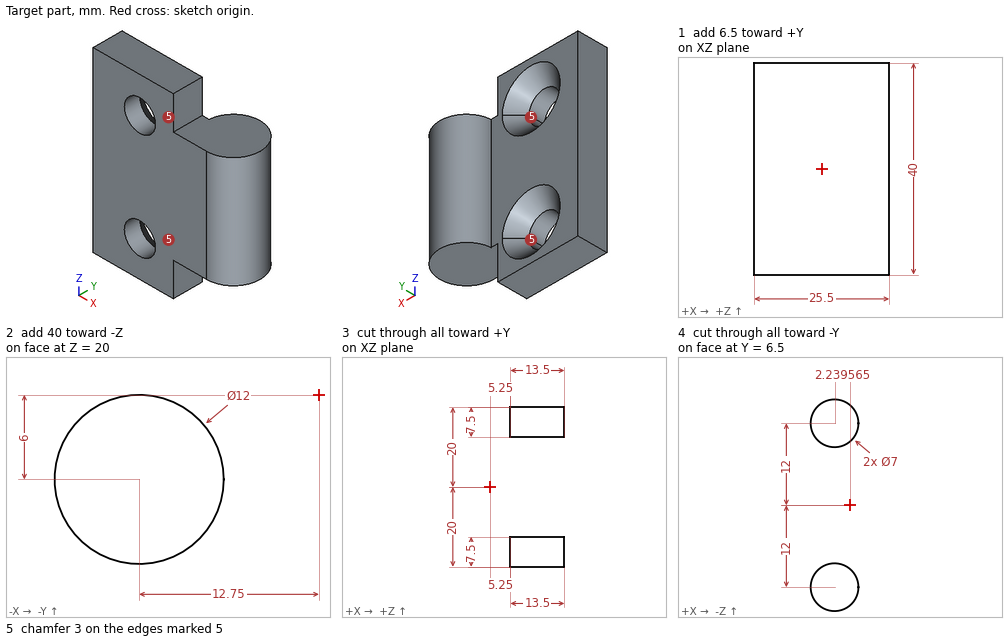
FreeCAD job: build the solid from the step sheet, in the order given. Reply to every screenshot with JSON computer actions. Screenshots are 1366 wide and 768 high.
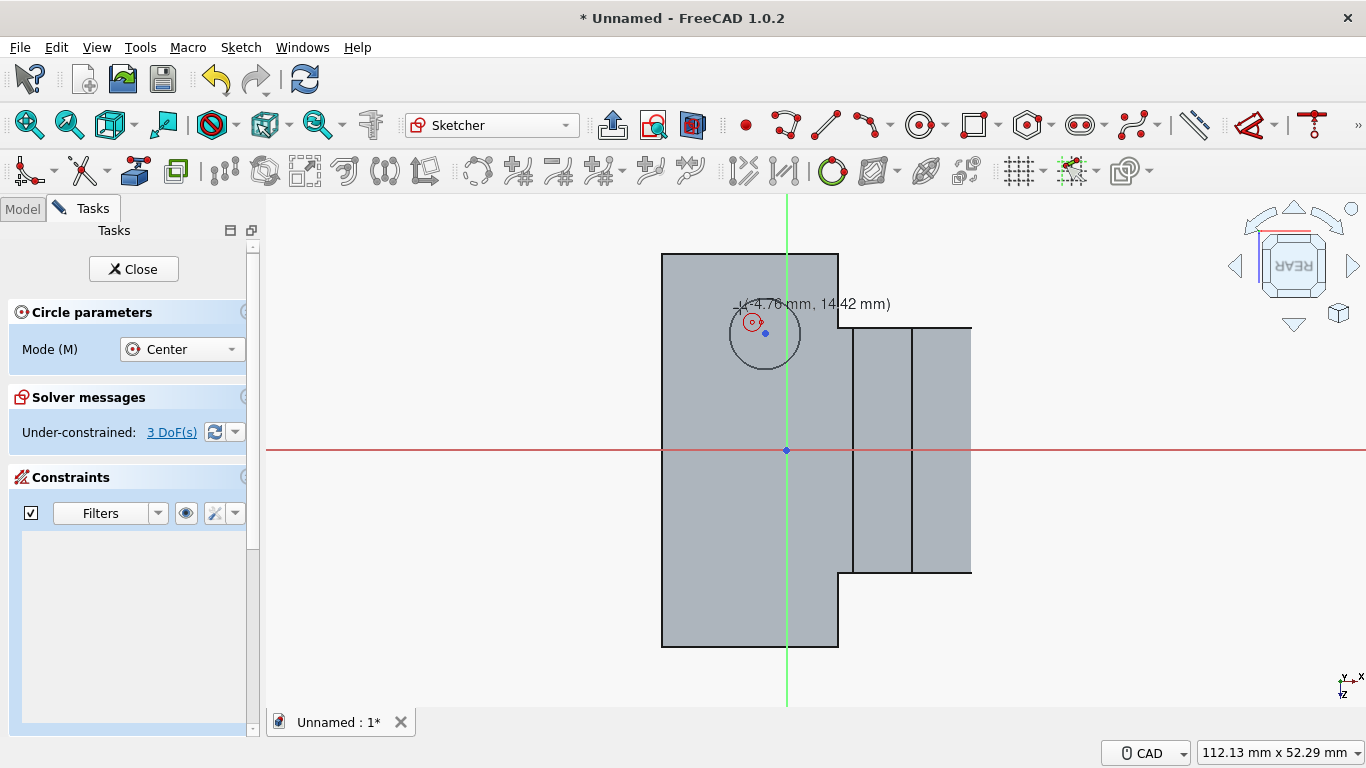
{"action": "left_click", "coordinate": [765, 568]}
{"action": "left_click", "coordinate": [740, 544]}
{"action": "key", "text": "Escape"}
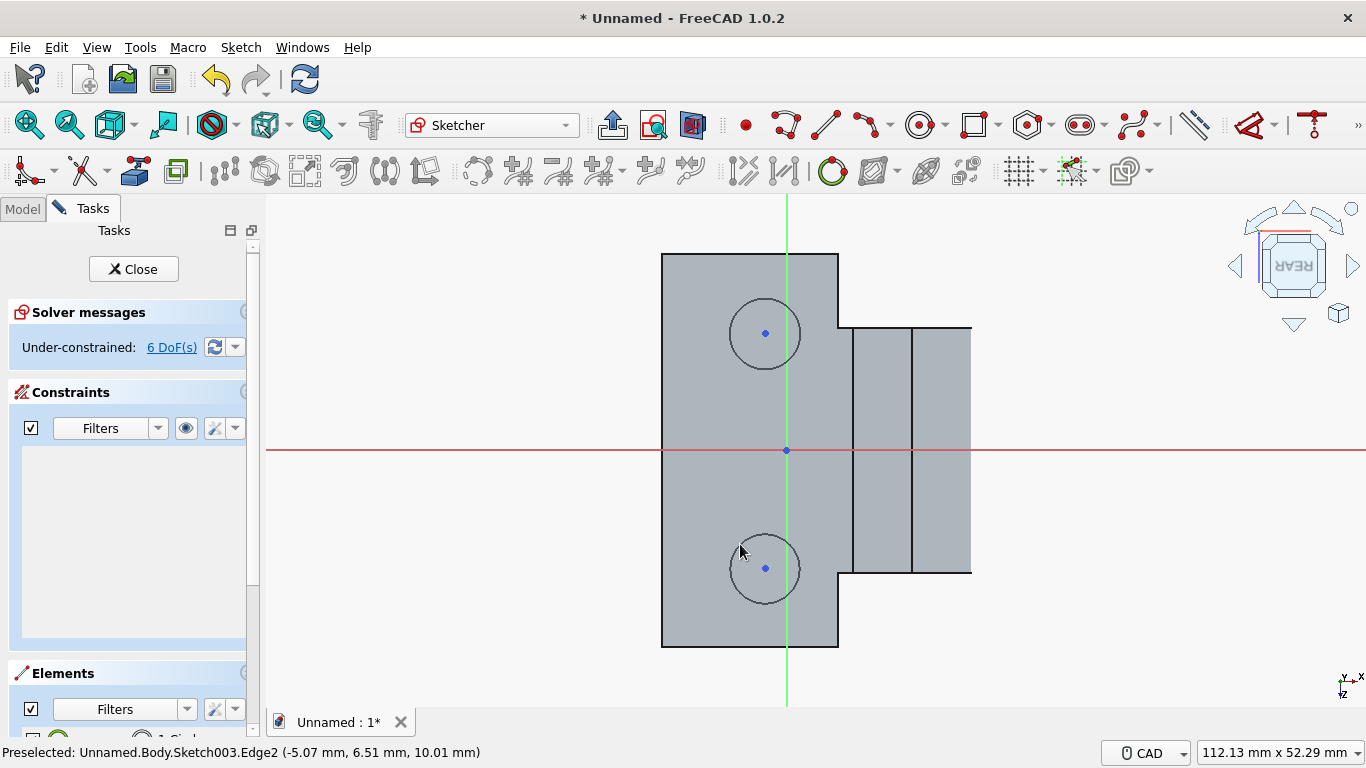
{"action": "left_click", "coordinate": [790, 309]}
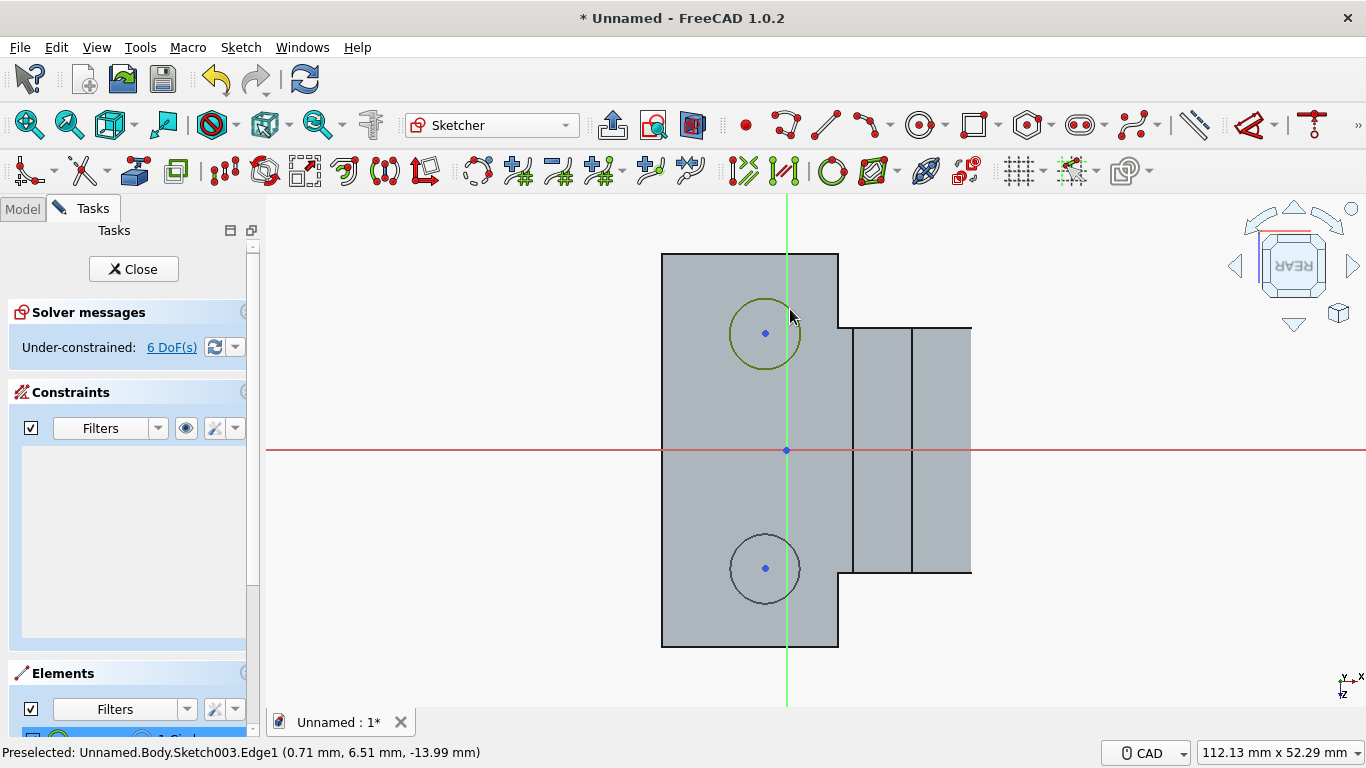
{"action": "left_click", "coordinate": [789, 544]}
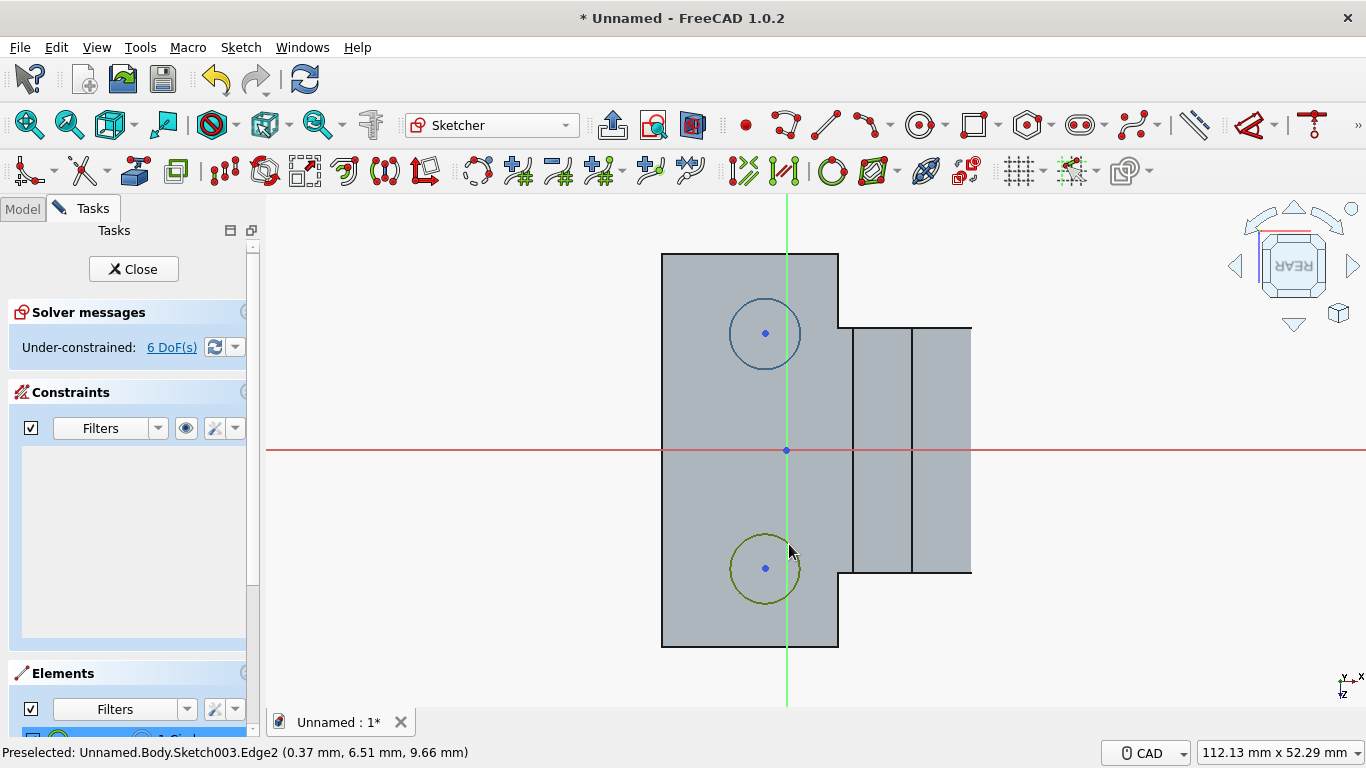
{"action": "key", "text": "e"}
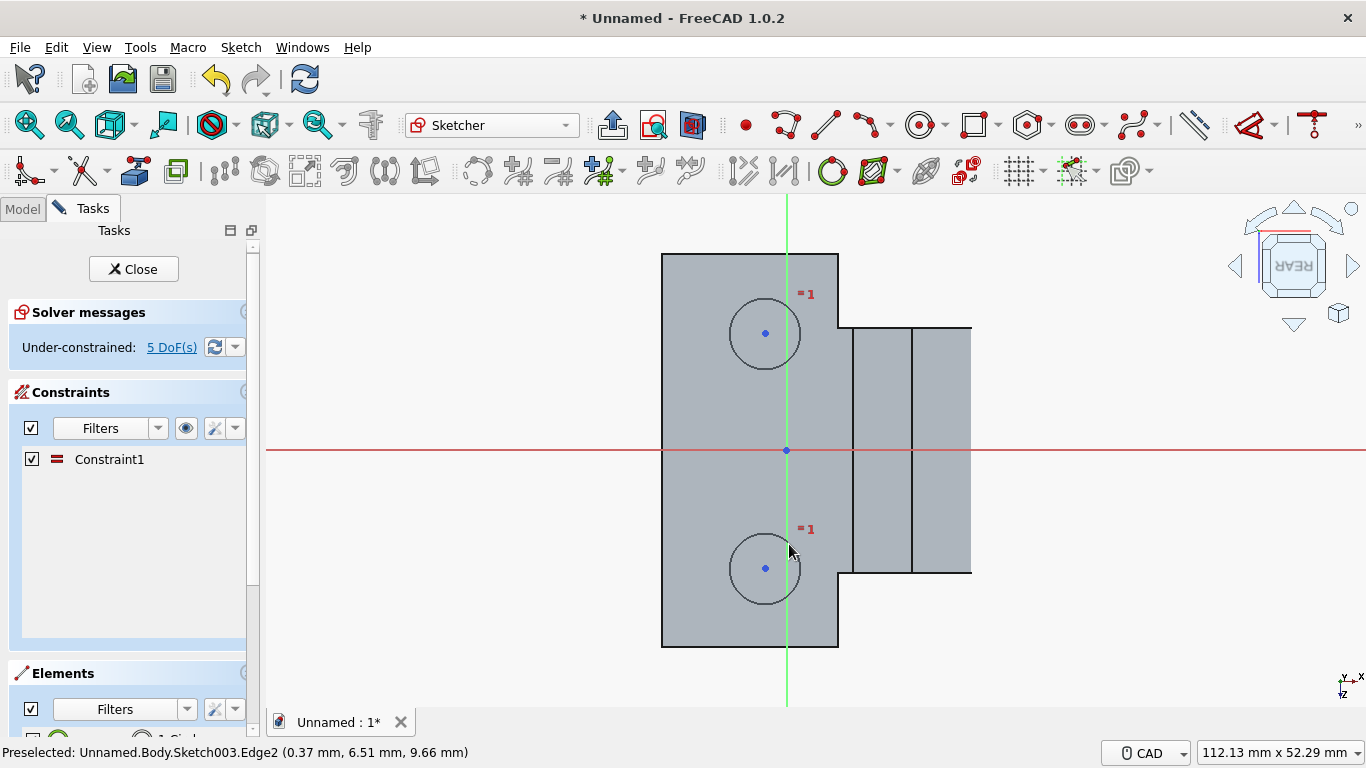
{"action": "left_click", "coordinate": [765, 334]}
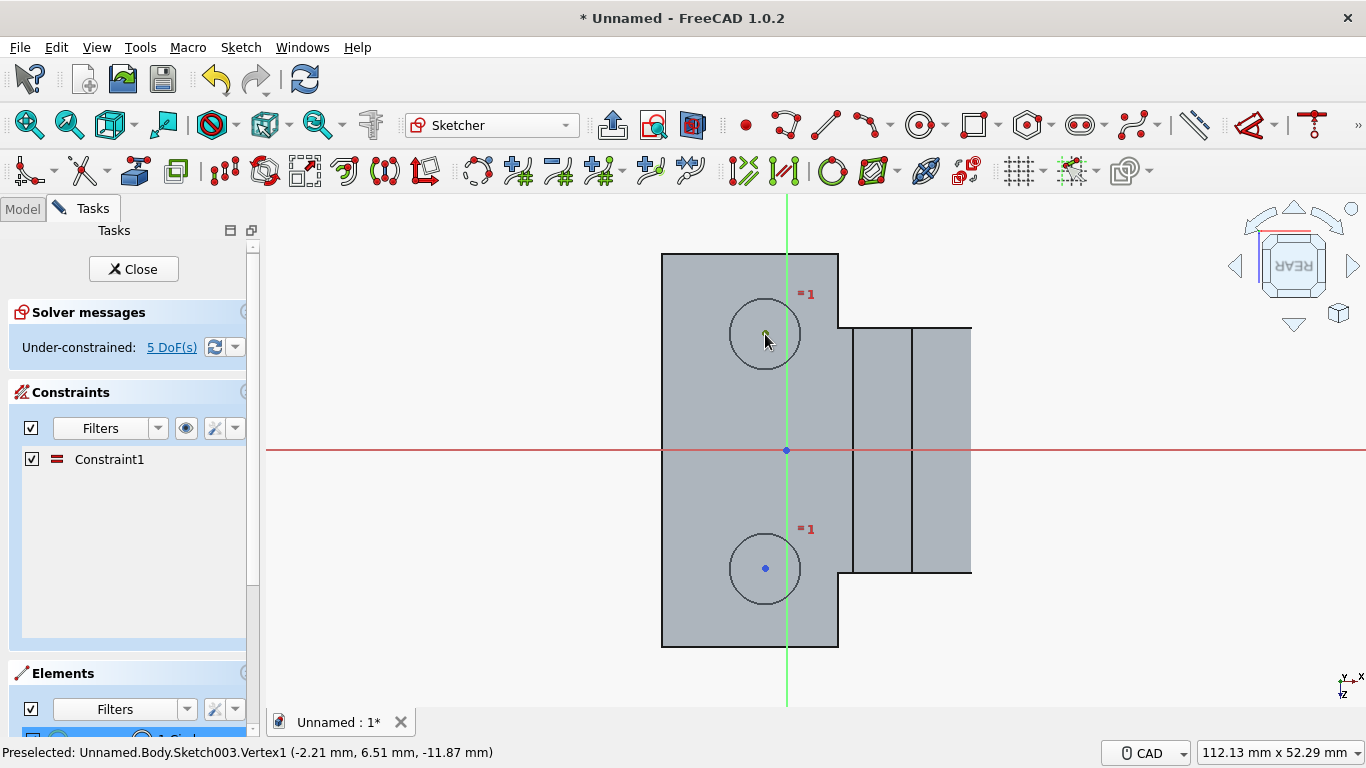
{"action": "left_click", "coordinate": [765, 569]}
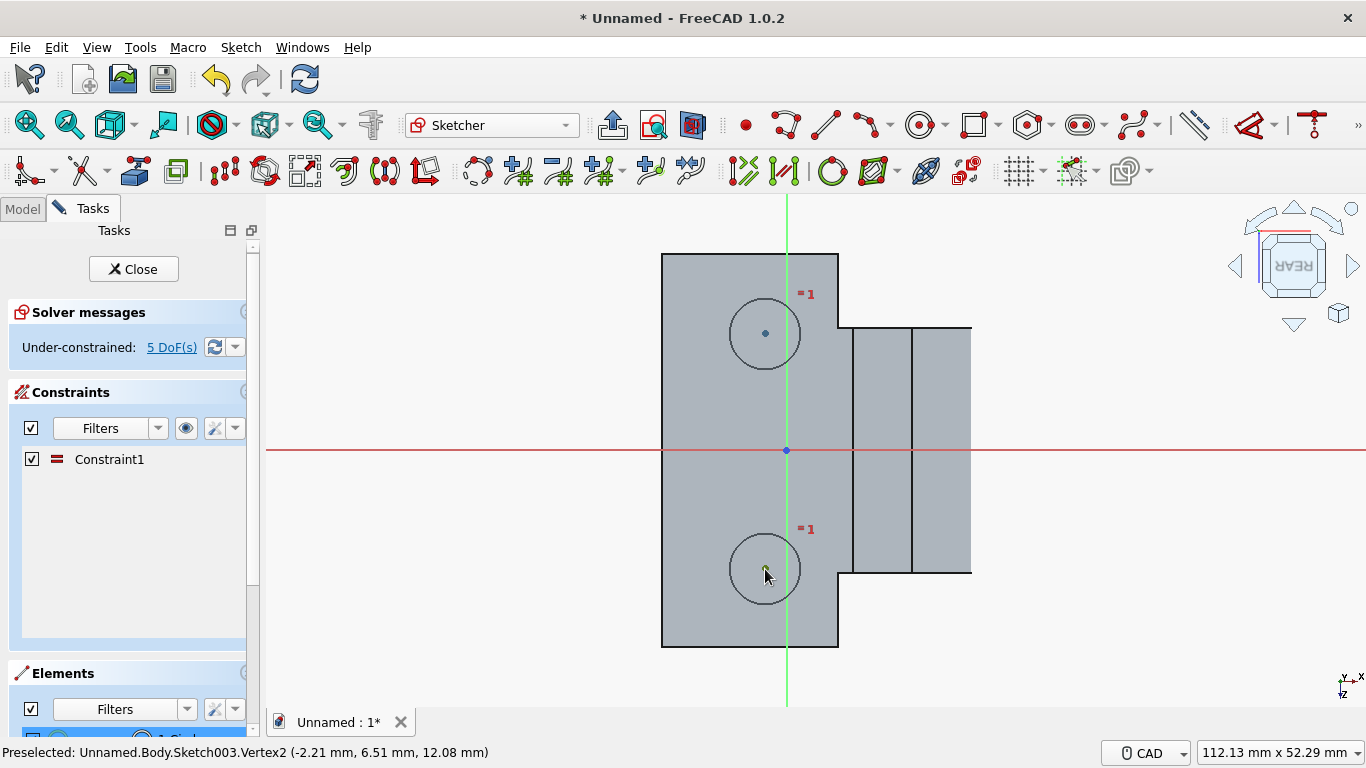
{"action": "key", "text": "v"}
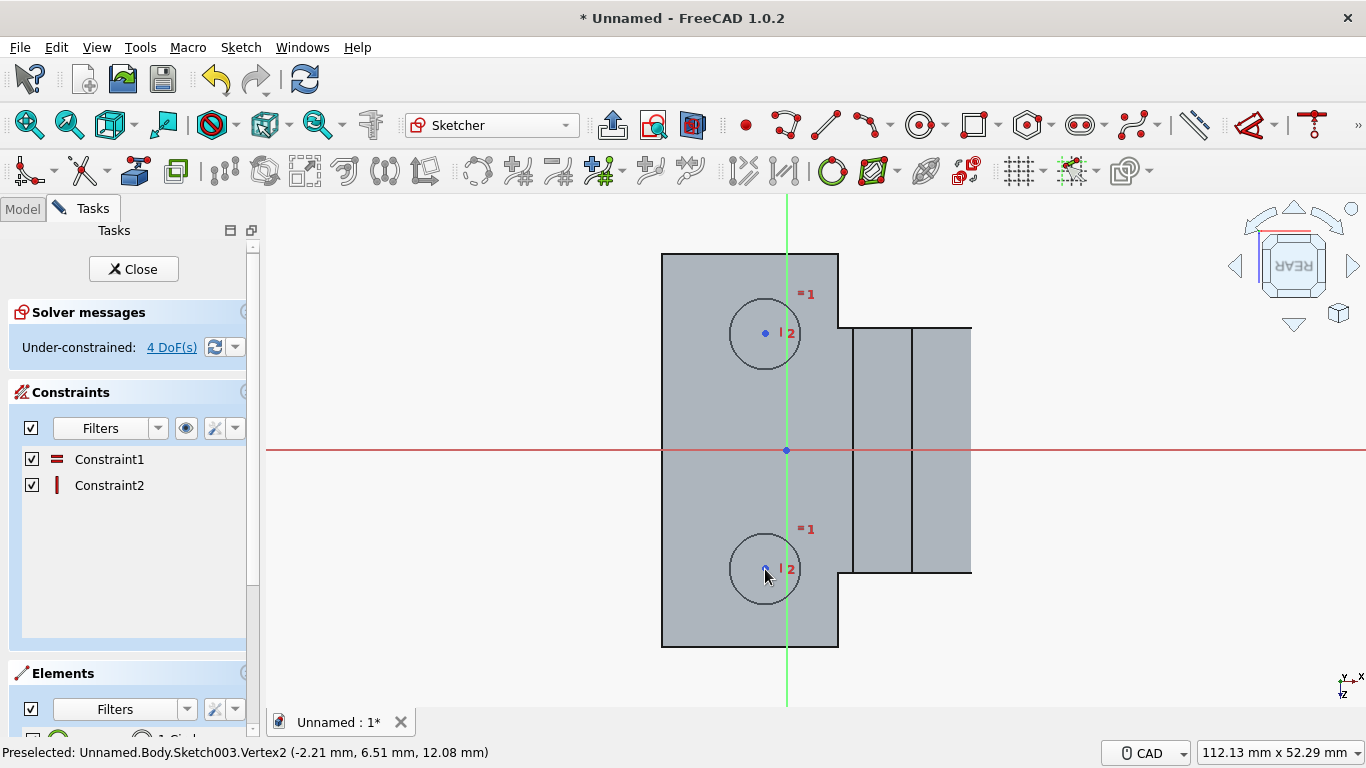
{"action": "key", "text": "d"}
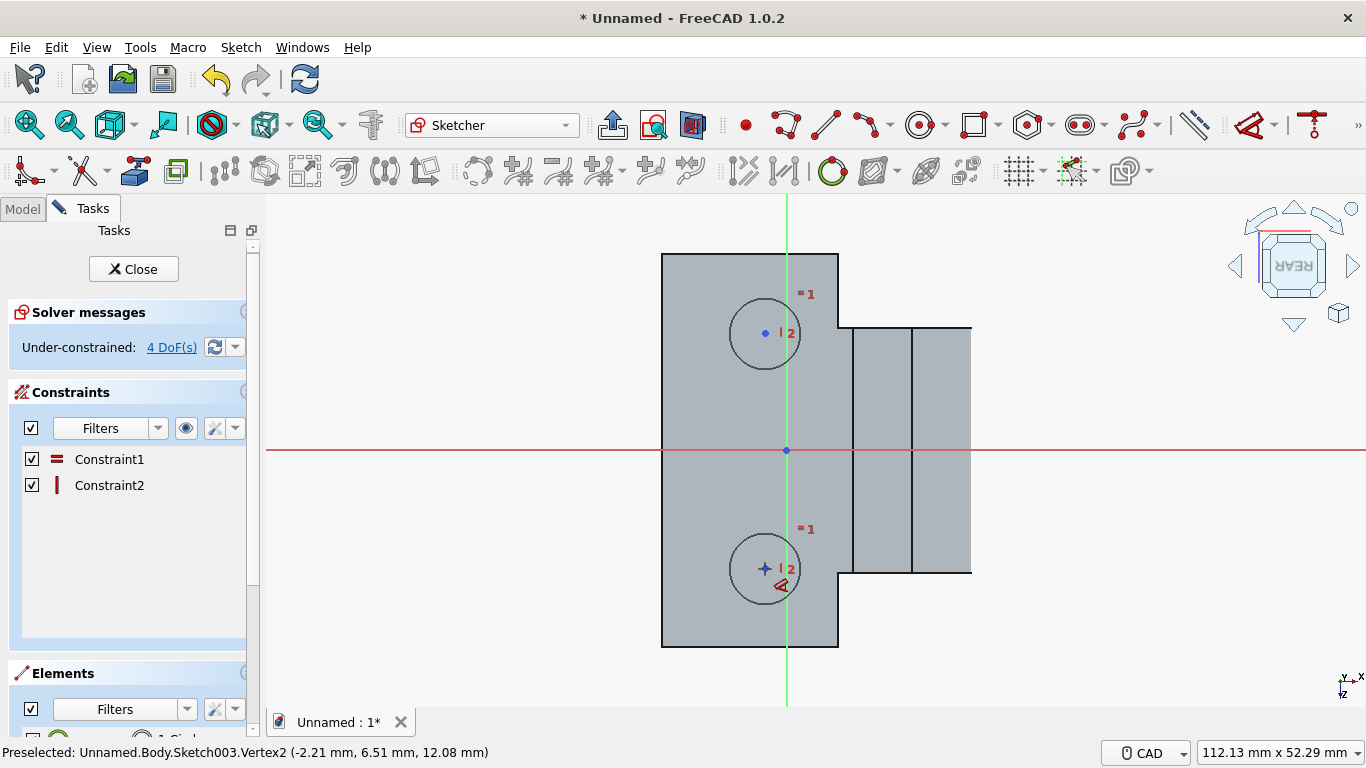
{"action": "left_click", "coordinate": [790, 309]}
{"action": "left_click", "coordinate": [813, 286]}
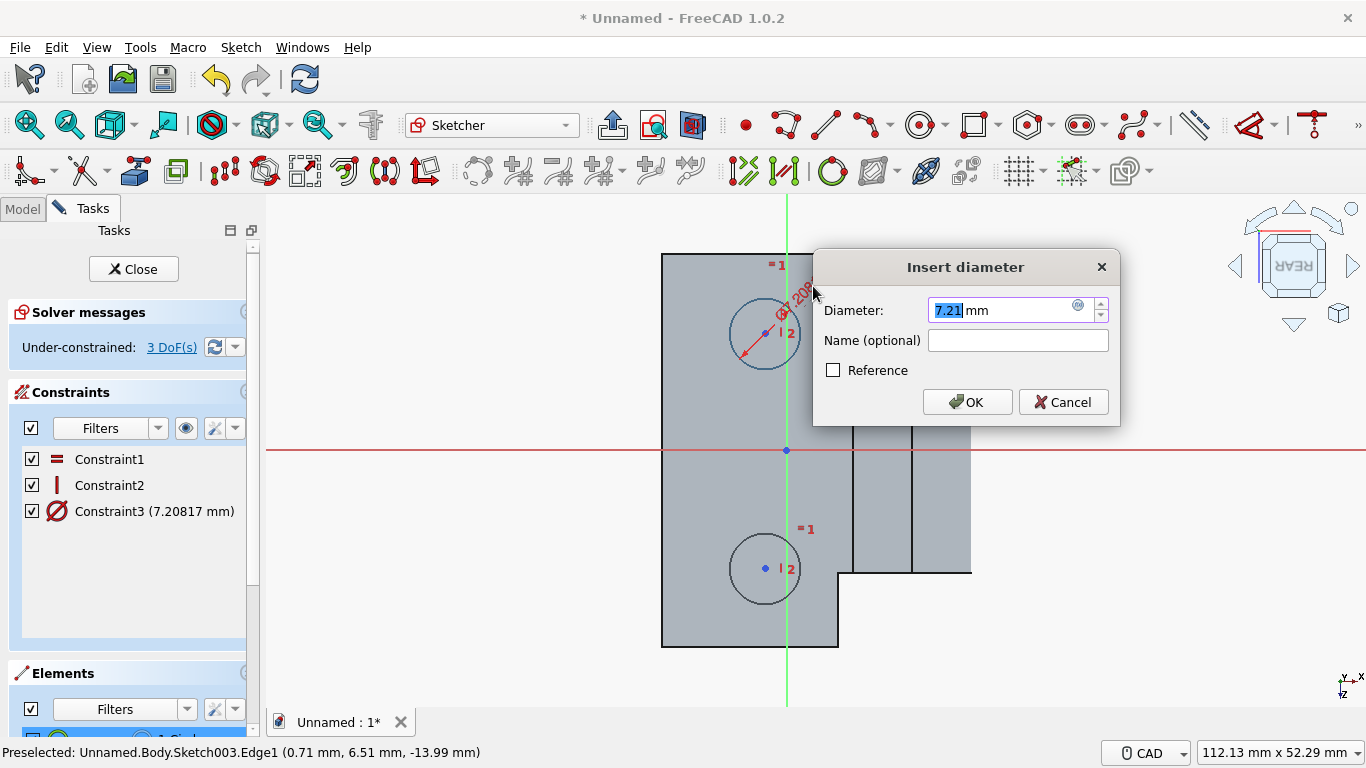
{"action": "type", "text": "7"}
{"action": "key", "text": "Return"}